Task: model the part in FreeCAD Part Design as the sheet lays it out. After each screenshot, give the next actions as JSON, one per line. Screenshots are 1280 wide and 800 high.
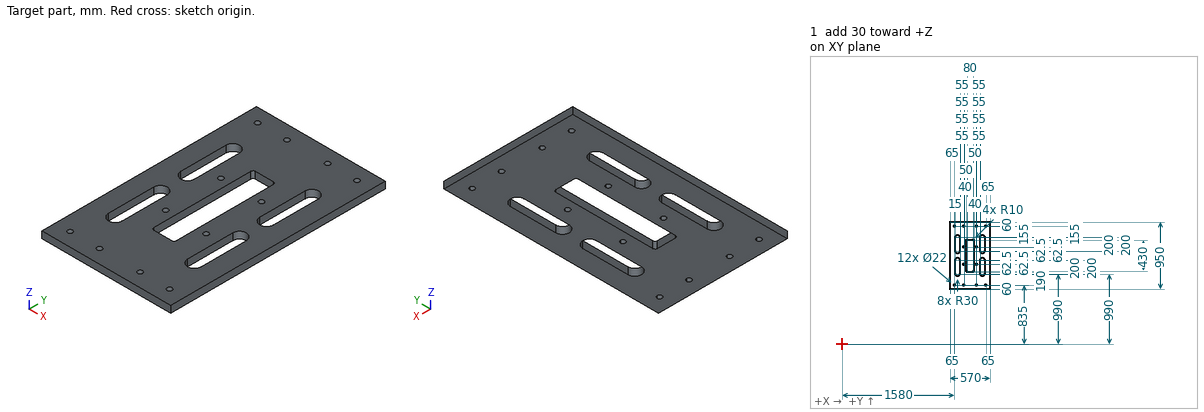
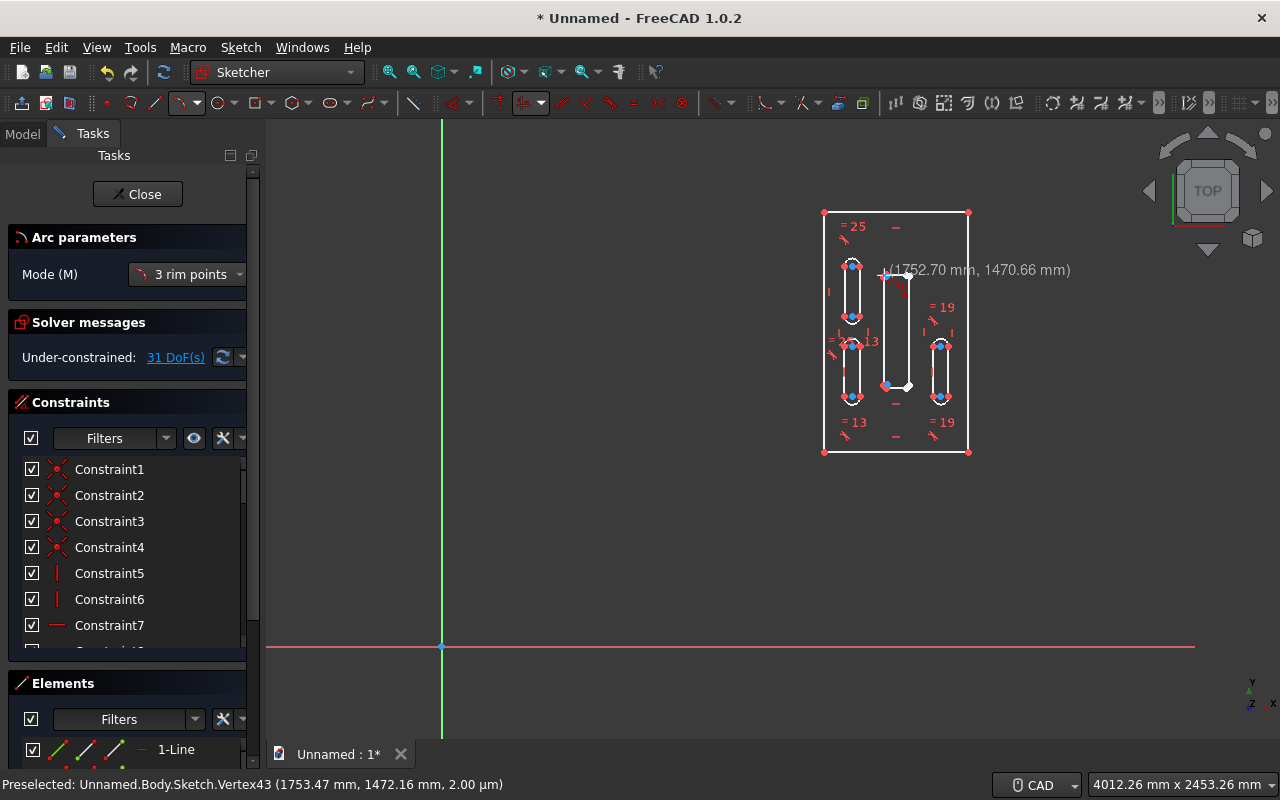
{"action": "scroll", "coordinate": [907, 274], "scroll_direction": "up", "scroll_amount": 8}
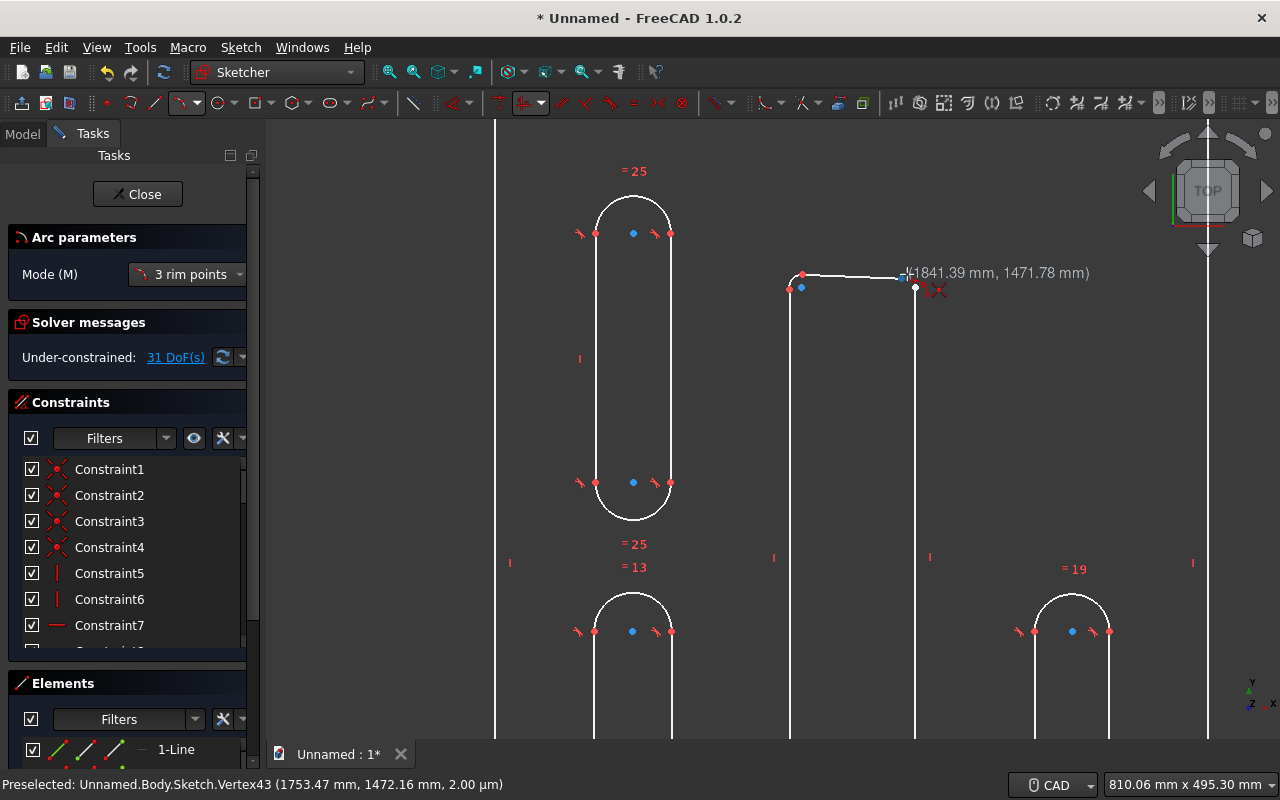
{"action": "left_click", "coordinate": [902, 279]}
{"action": "left_click", "coordinate": [915, 288]}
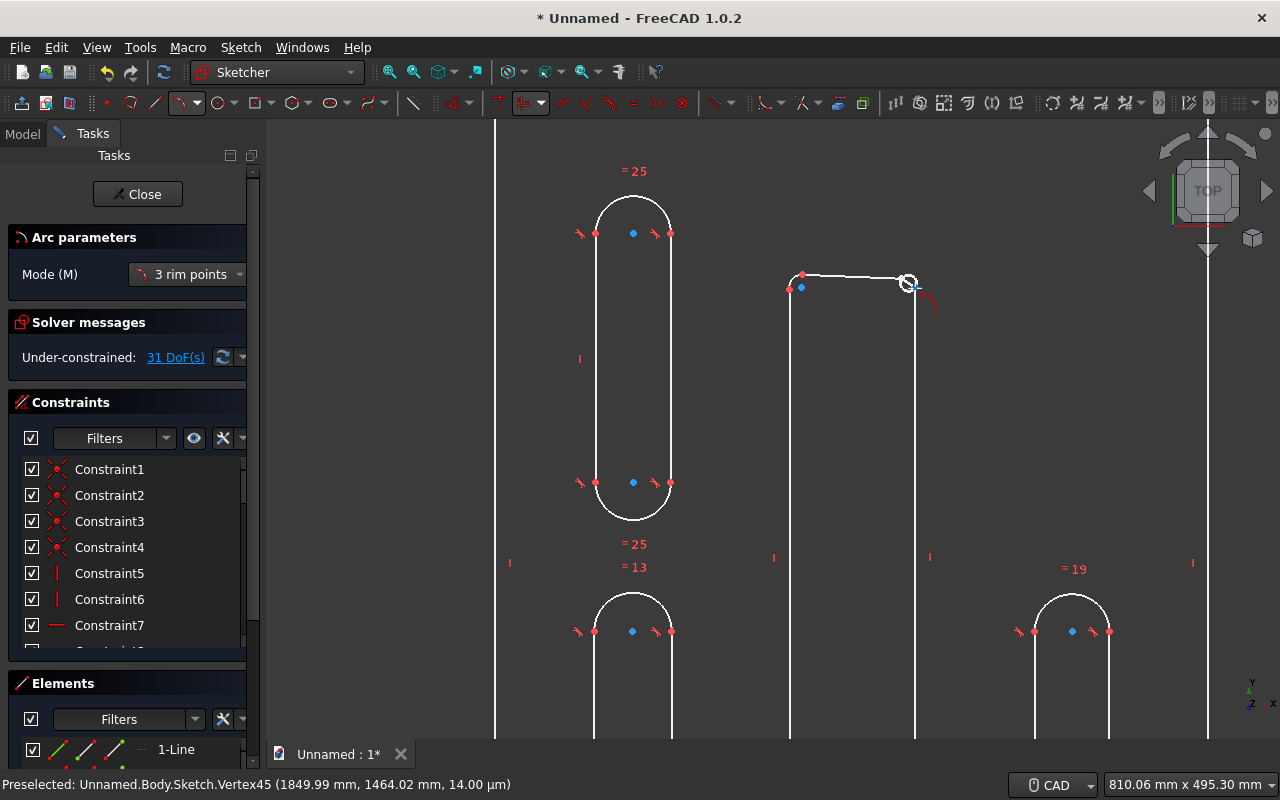
{"action": "scroll", "coordinate": [912, 278], "scroll_direction": "up", "scroll_amount": 8}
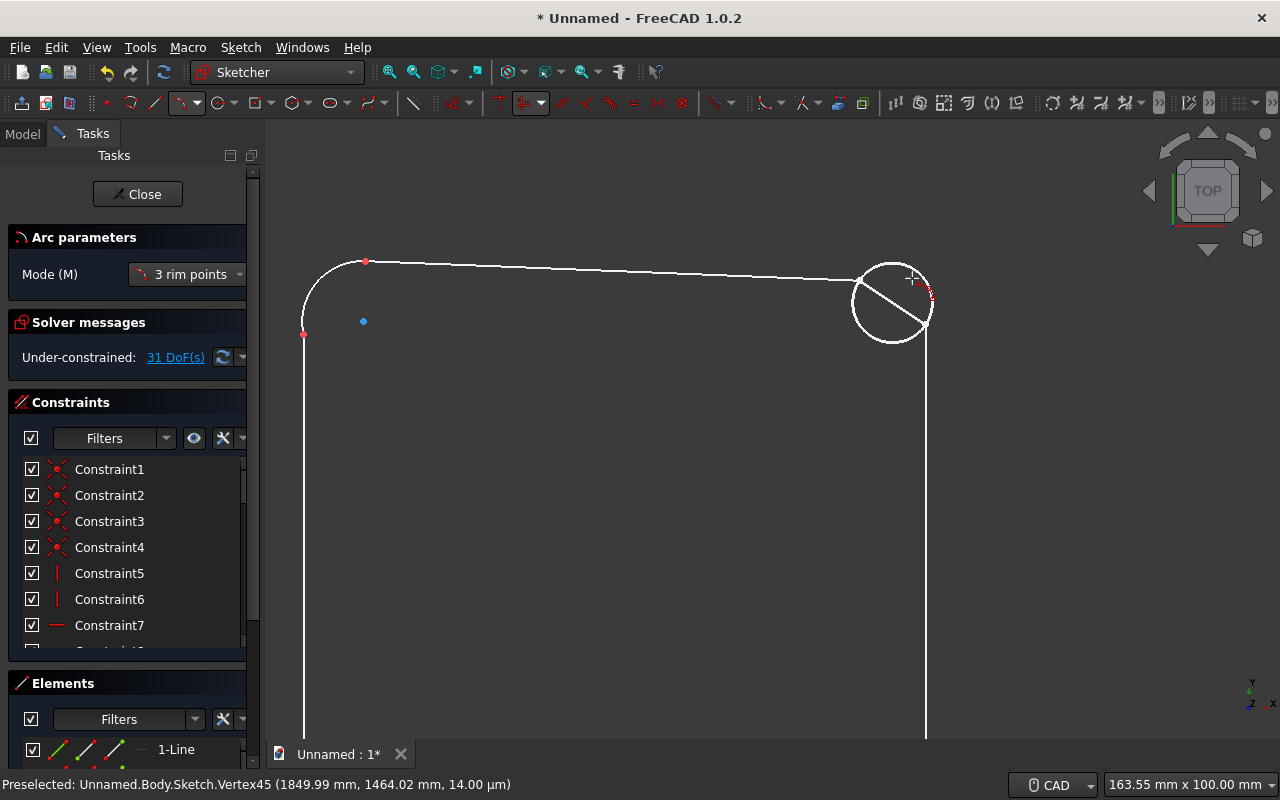
{"action": "left_click", "coordinate": [908, 275]}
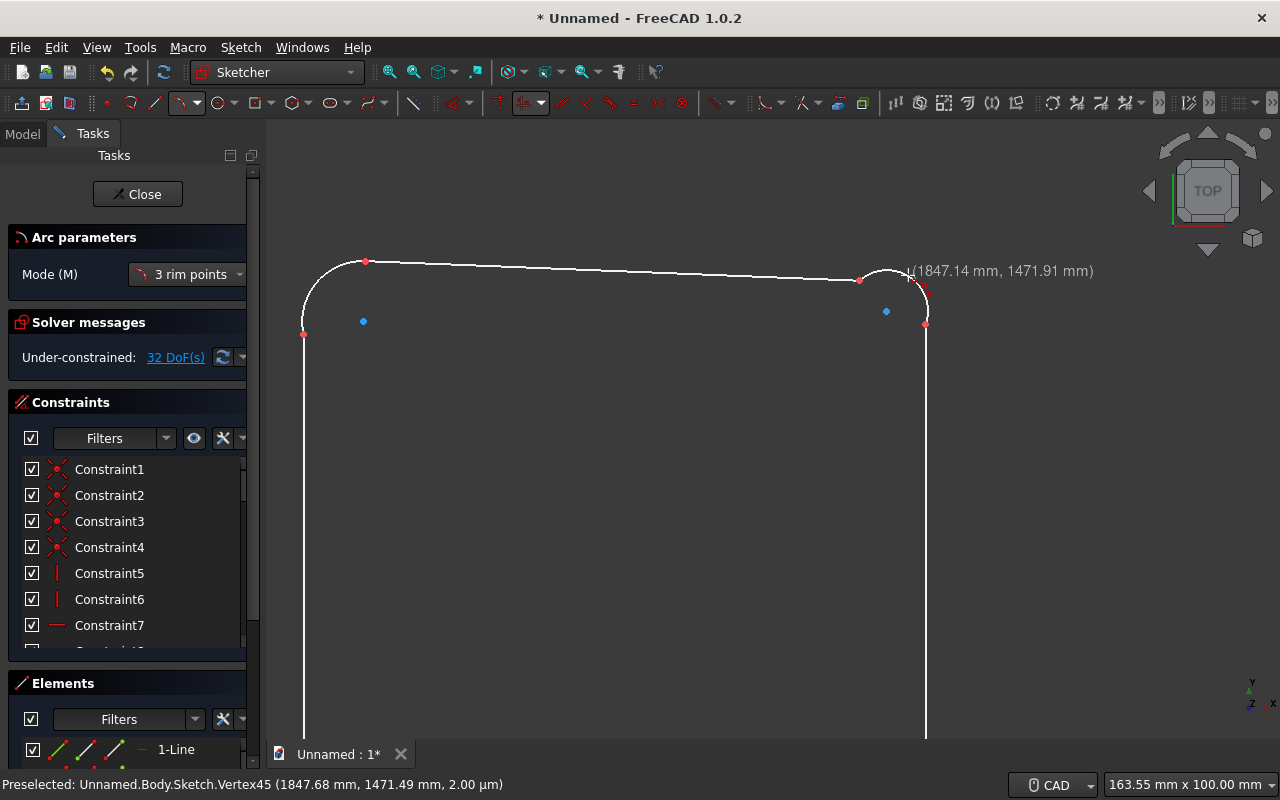
{"action": "scroll", "coordinate": [908, 275], "scroll_direction": "down", "scroll_amount": 16}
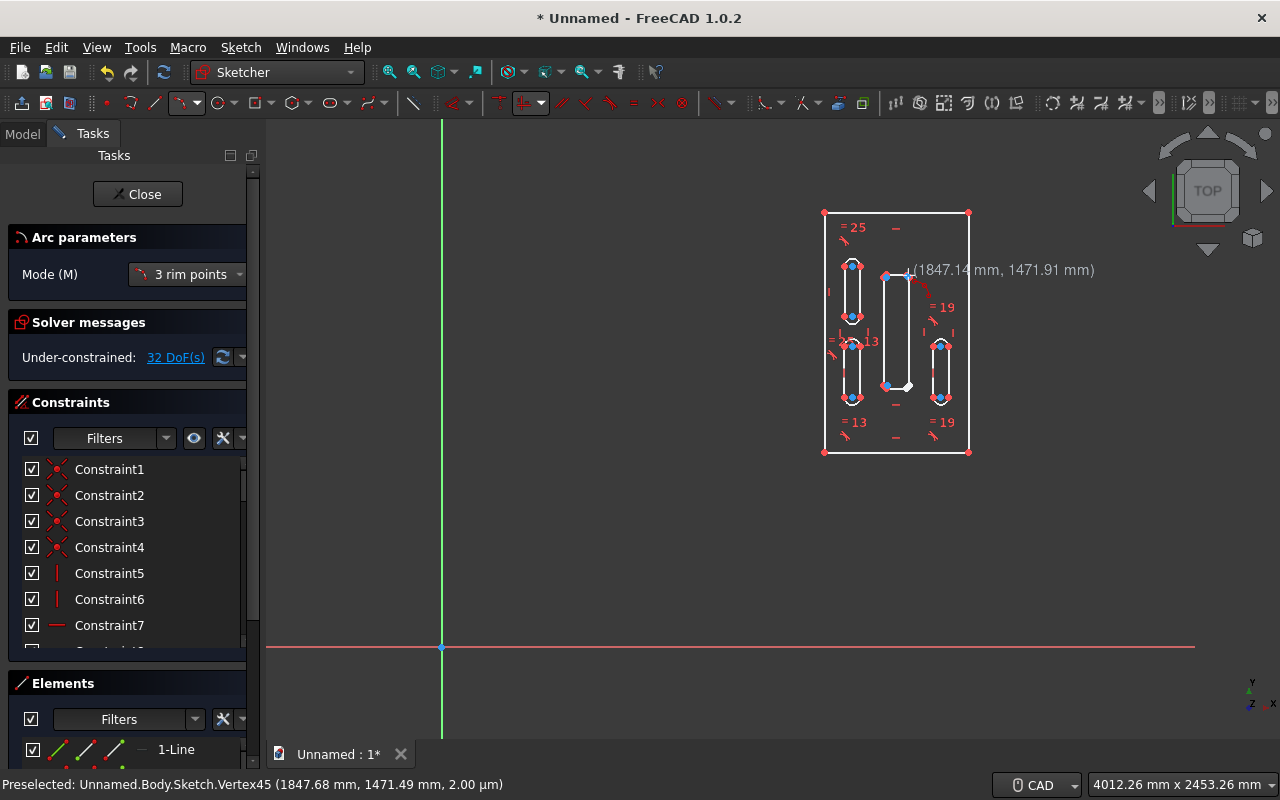
{"action": "scroll", "coordinate": [909, 386], "scroll_direction": "up", "scroll_amount": 8}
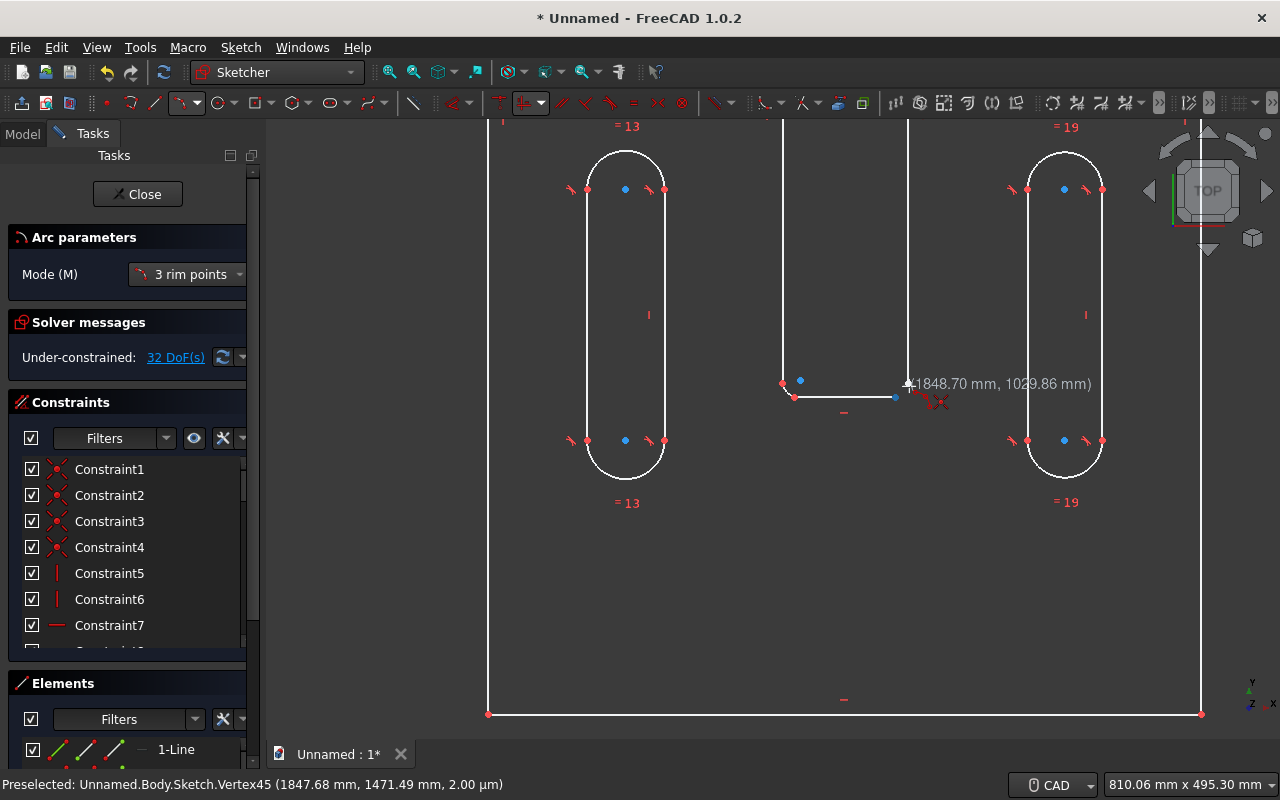
{"action": "left_click", "coordinate": [908, 383]}
{"action": "left_click", "coordinate": [895, 397]}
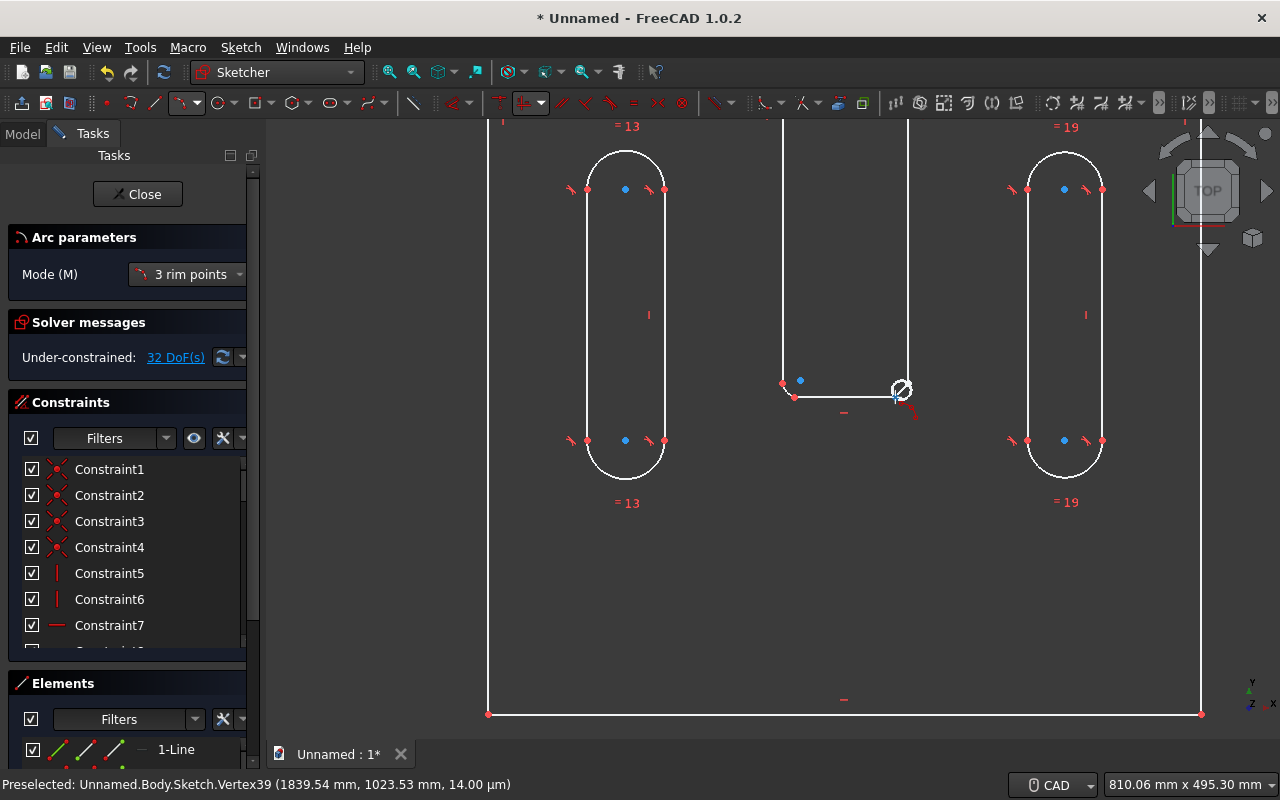
{"action": "scroll", "coordinate": [904, 392], "scroll_direction": "up", "scroll_amount": 8}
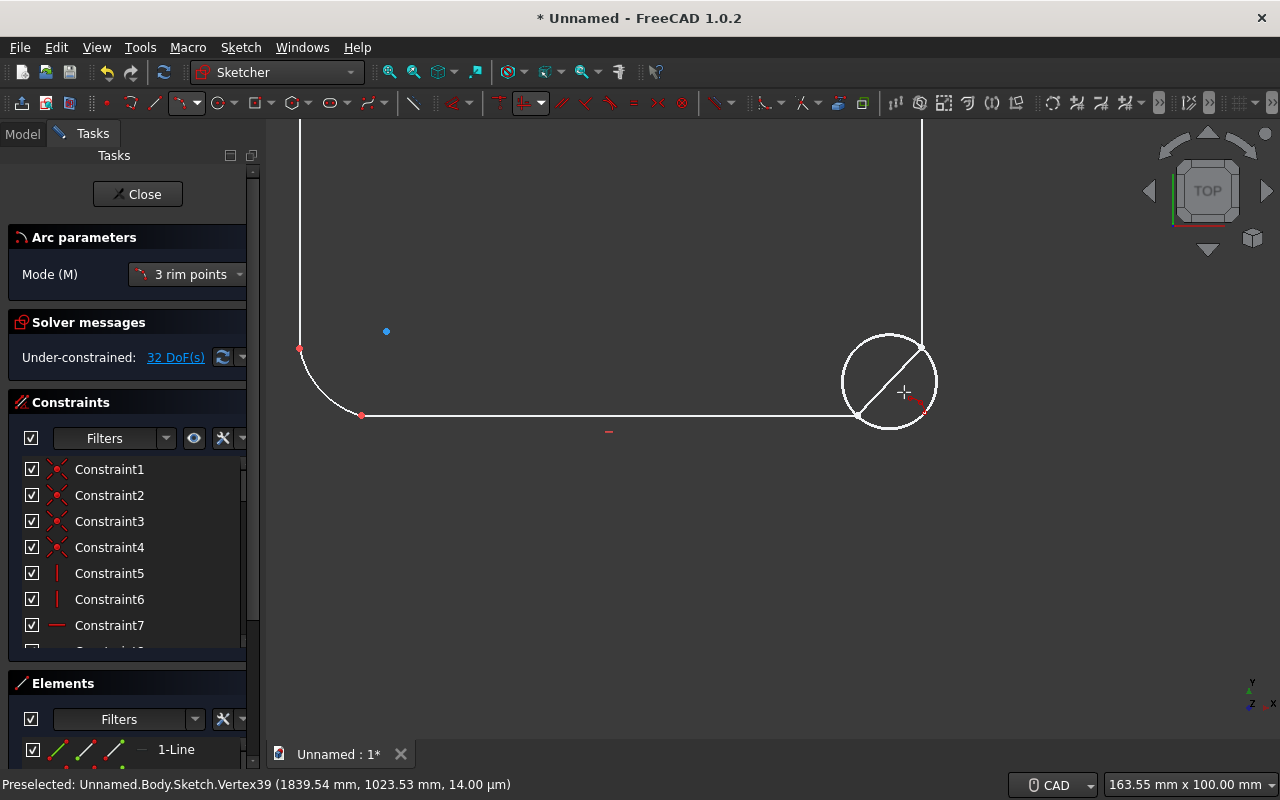
{"action": "left_click", "coordinate": [904, 389]}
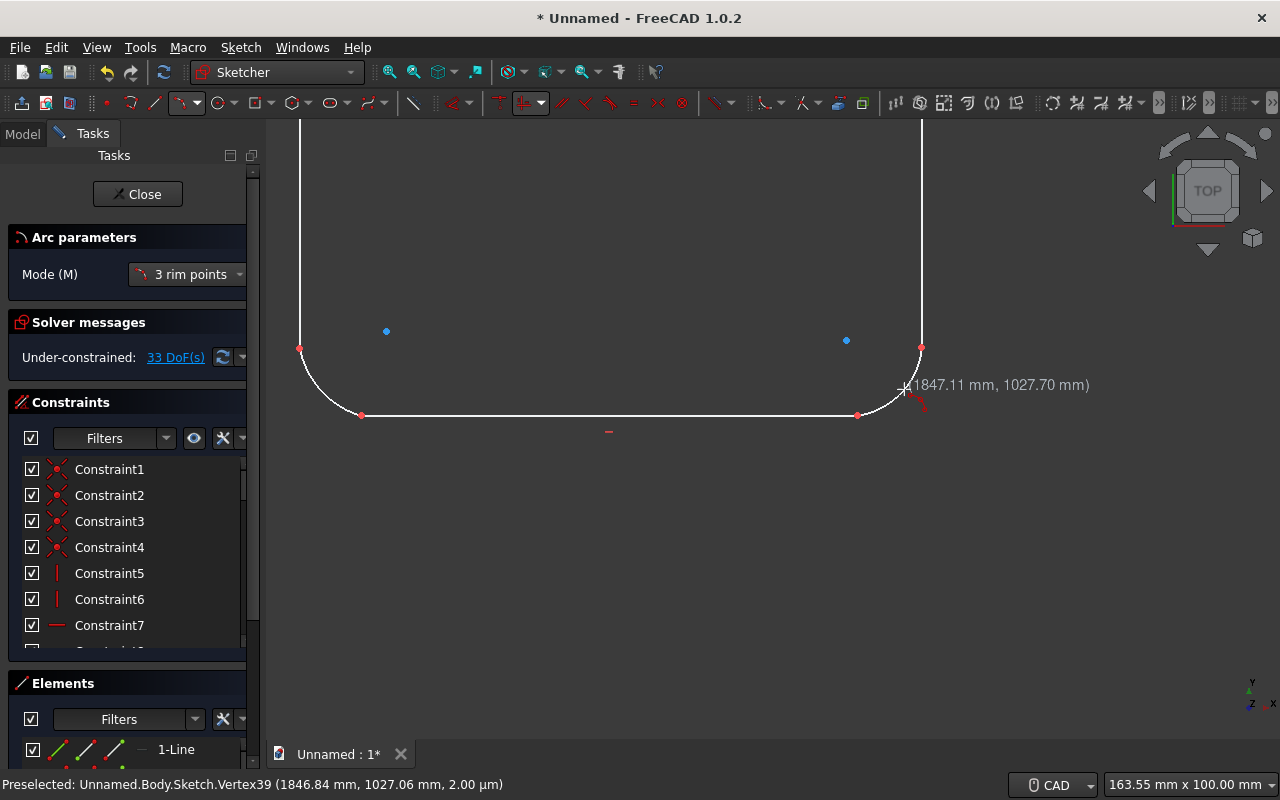
{"action": "left_click", "coordinate": [330, 104]}